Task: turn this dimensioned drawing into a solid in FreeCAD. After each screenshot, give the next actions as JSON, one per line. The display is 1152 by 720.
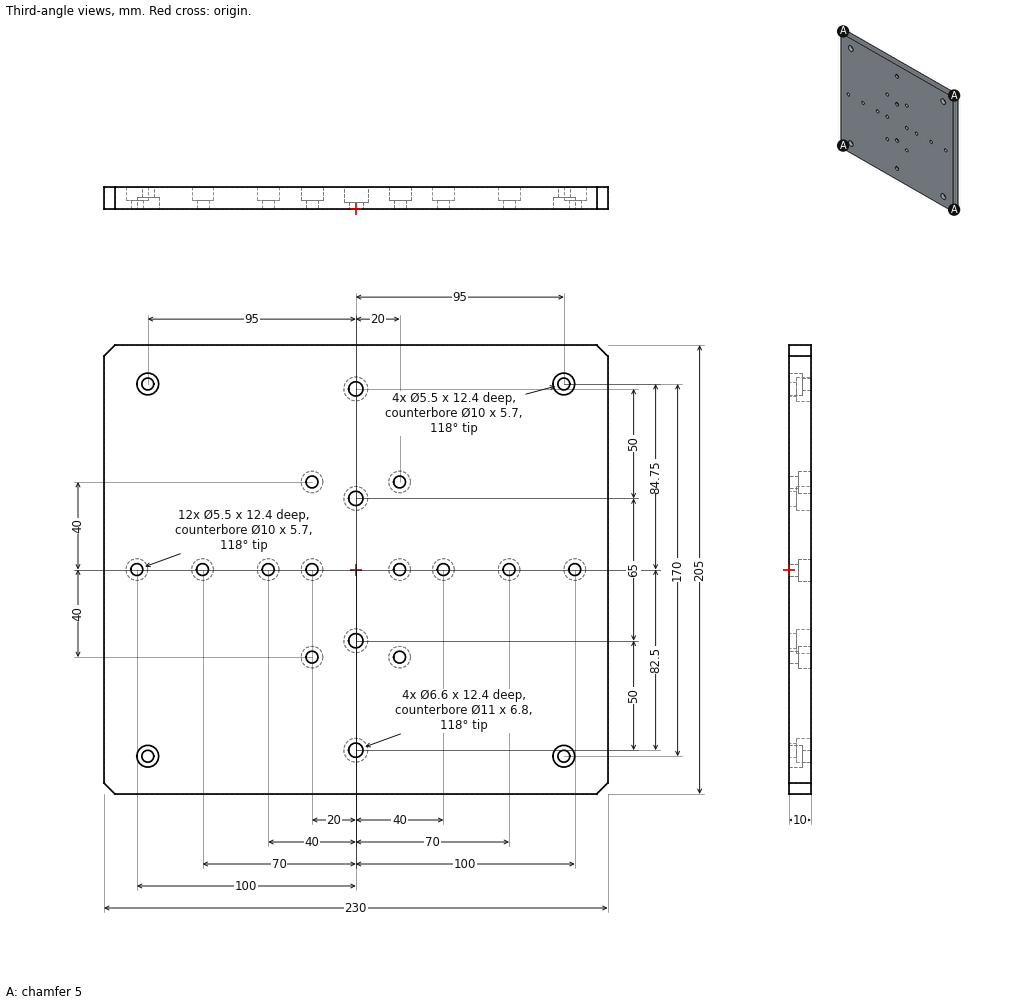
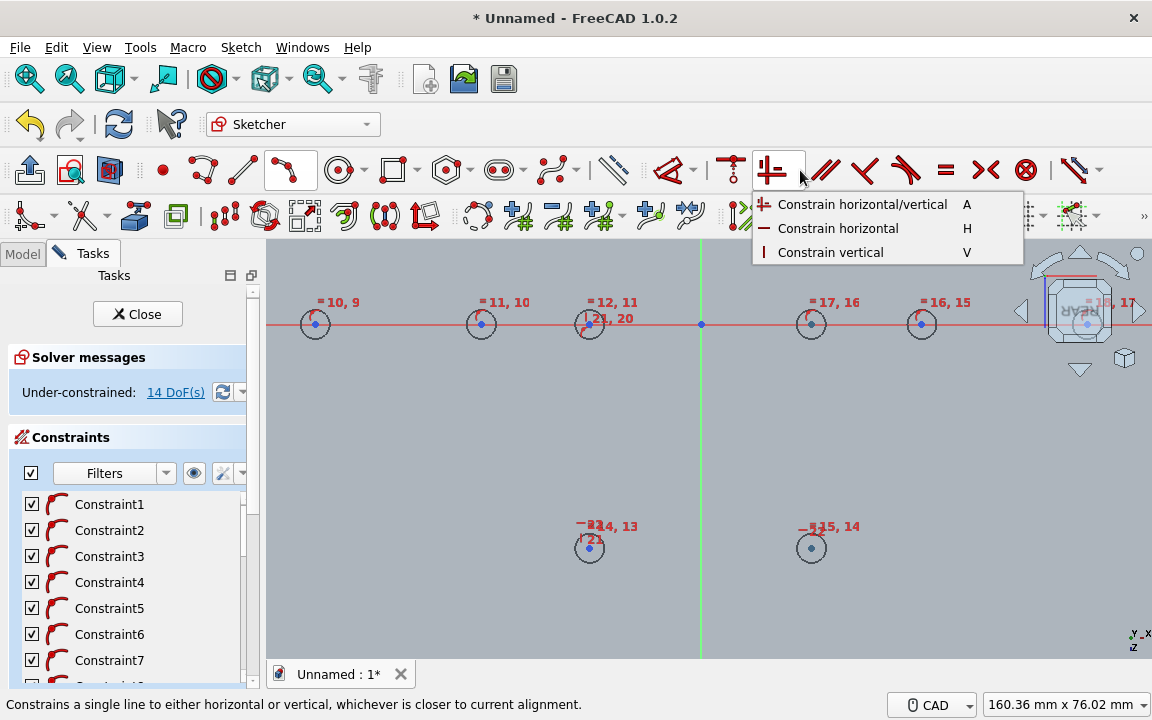
{"action": "left_click", "coordinate": [888, 252]}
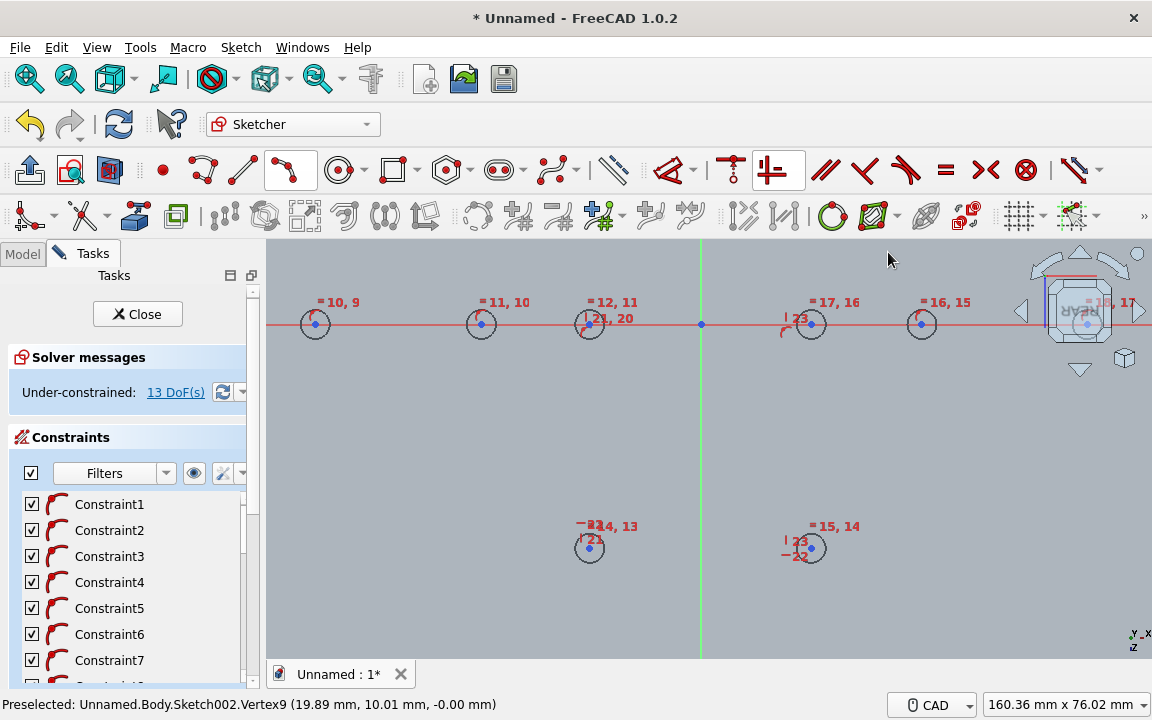
{"action": "left_click", "coordinate": [811, 325]}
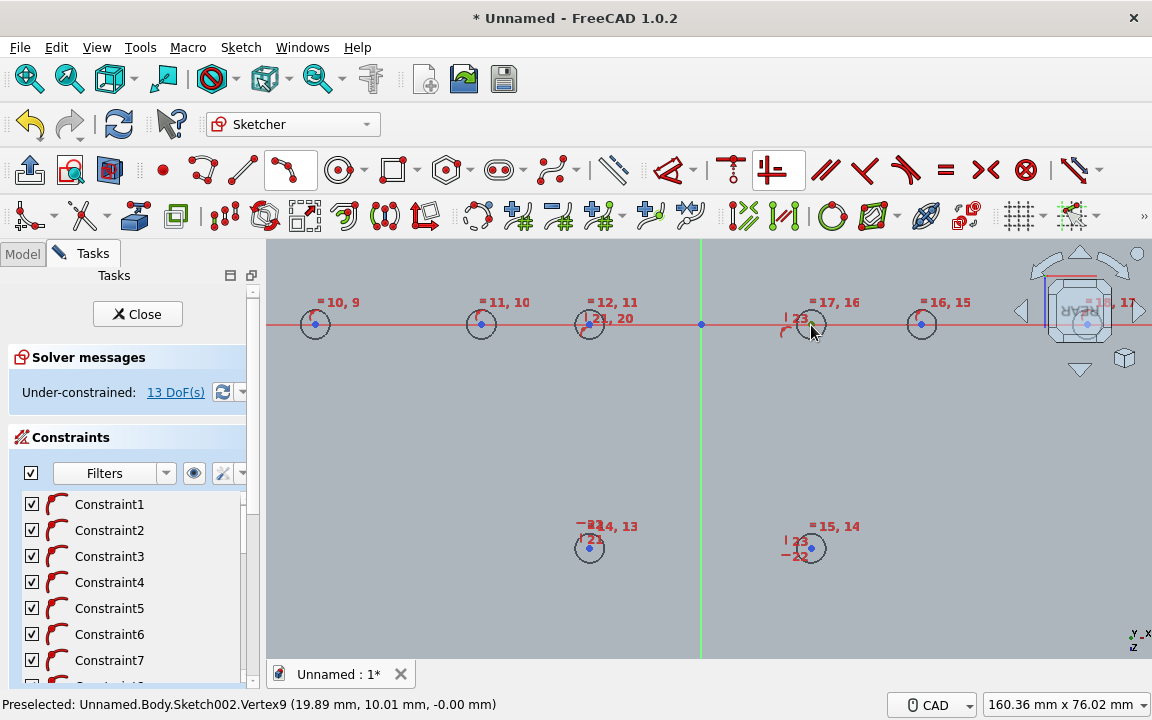
{"action": "scroll", "coordinate": [591, 551], "scroll_direction": "down", "scroll_amount": 4}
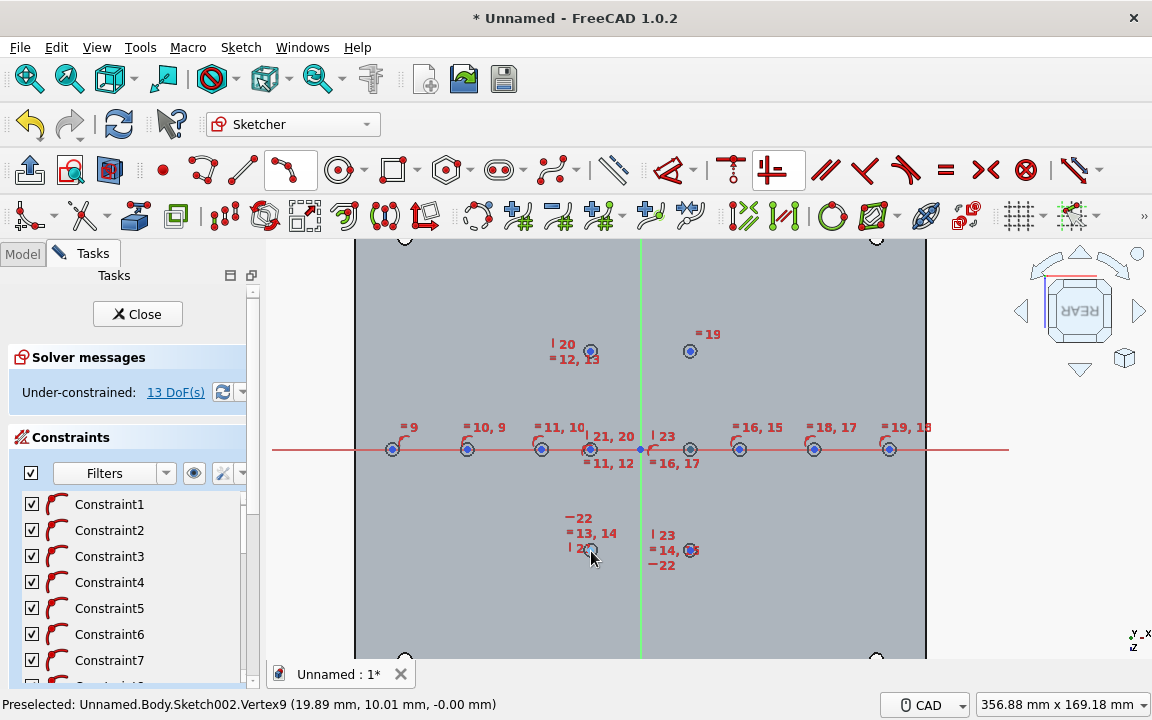
{"action": "left_click", "coordinate": [690, 351]}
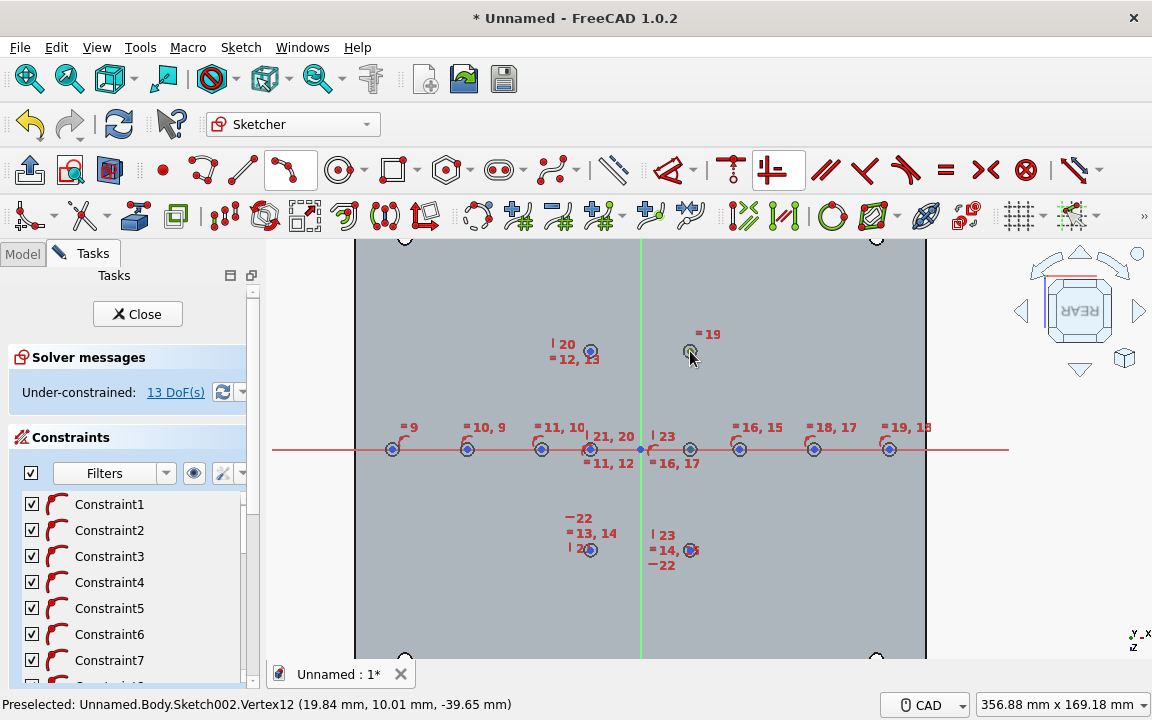
{"action": "key", "text": "v"}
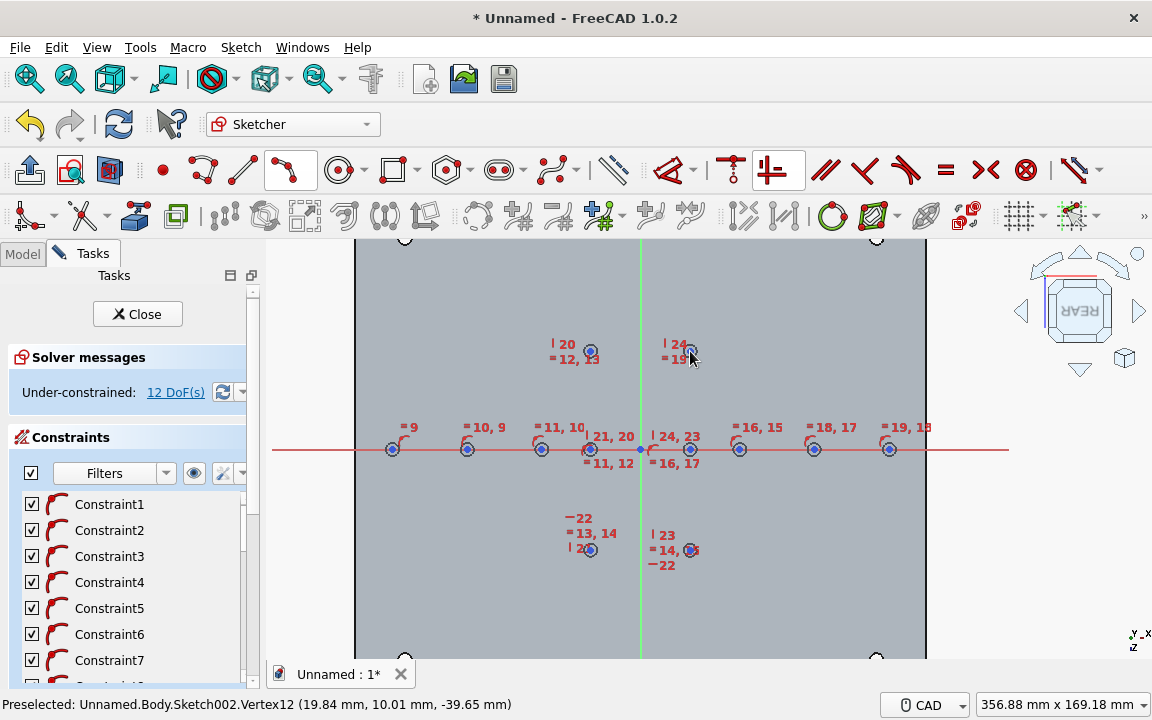
{"action": "scroll", "coordinate": [591, 351], "scroll_direction": "up", "scroll_amount": 4}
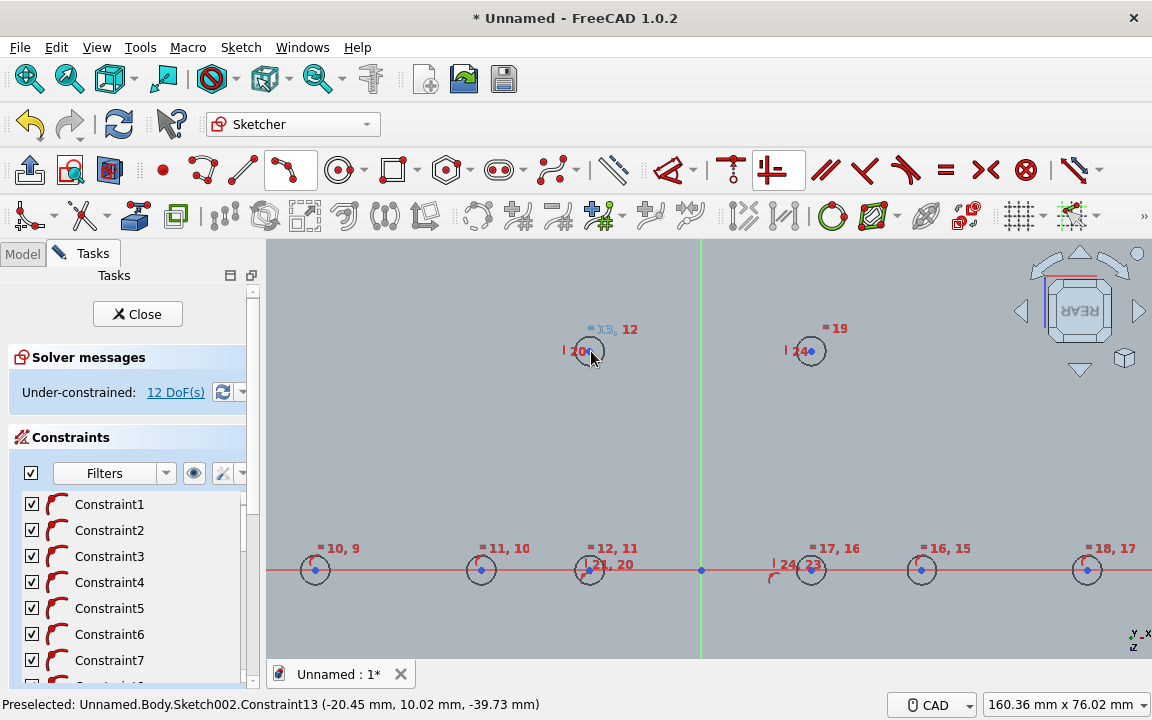
{"action": "left_click", "coordinate": [590, 351]}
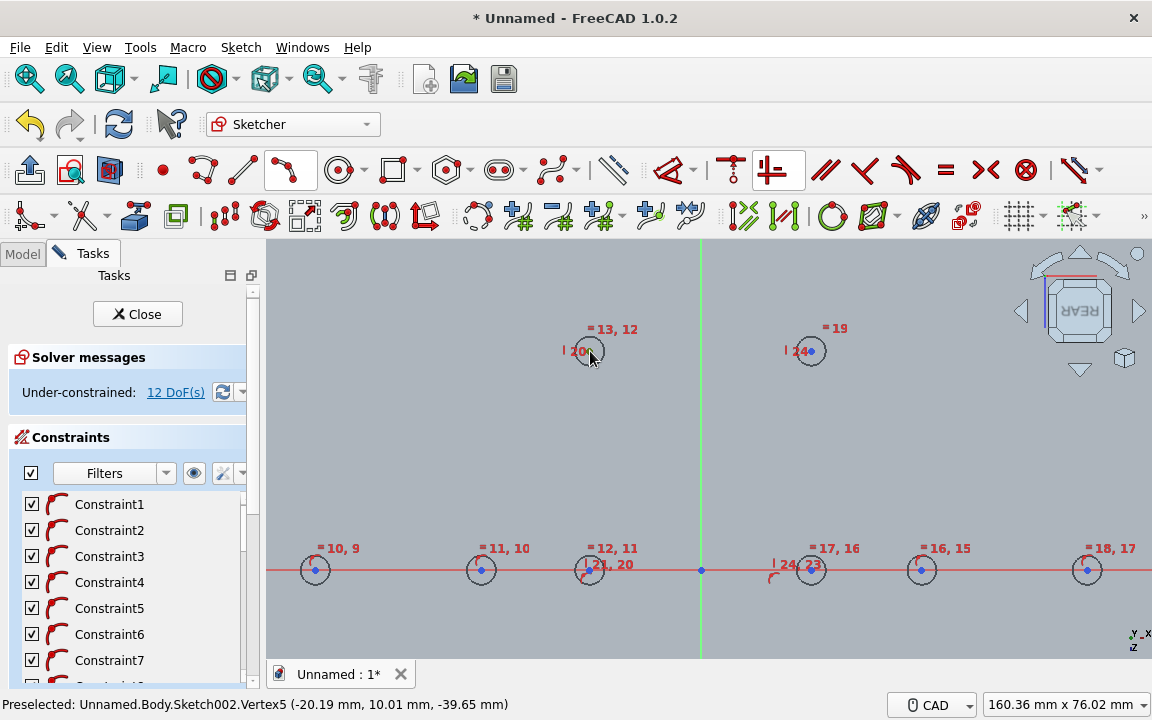
{"action": "left_click", "coordinate": [811, 351]}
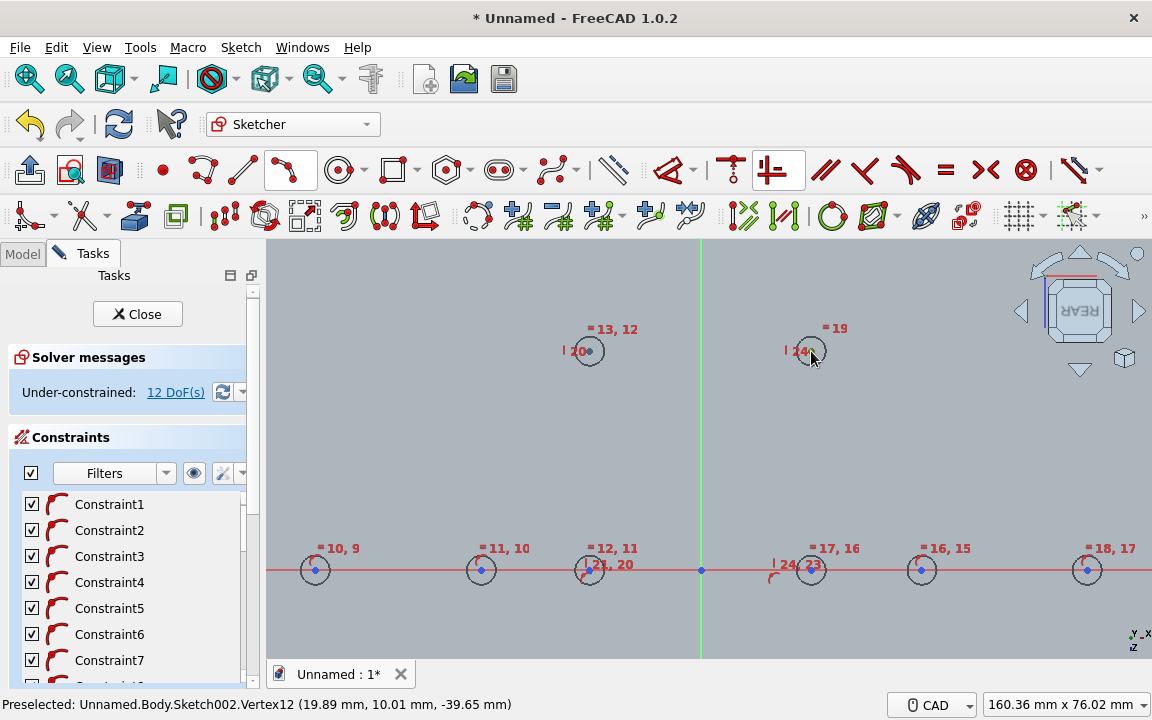
{"action": "key", "text": "h"}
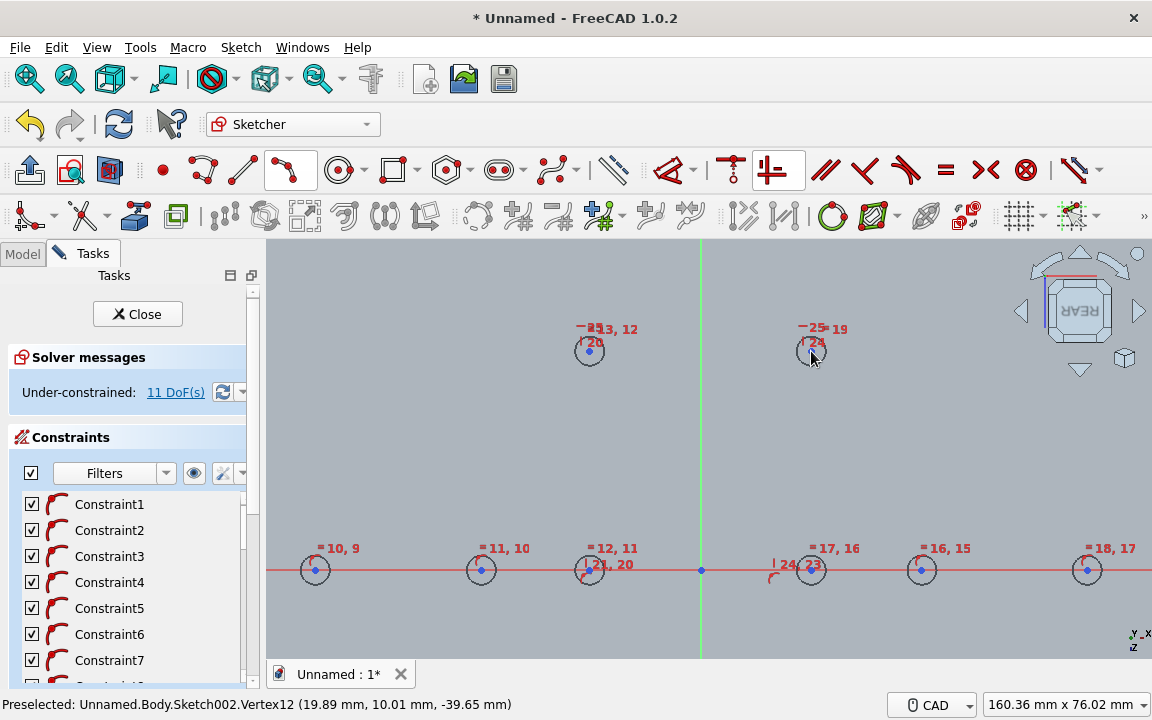
{"action": "left_click", "coordinate": [668, 170]}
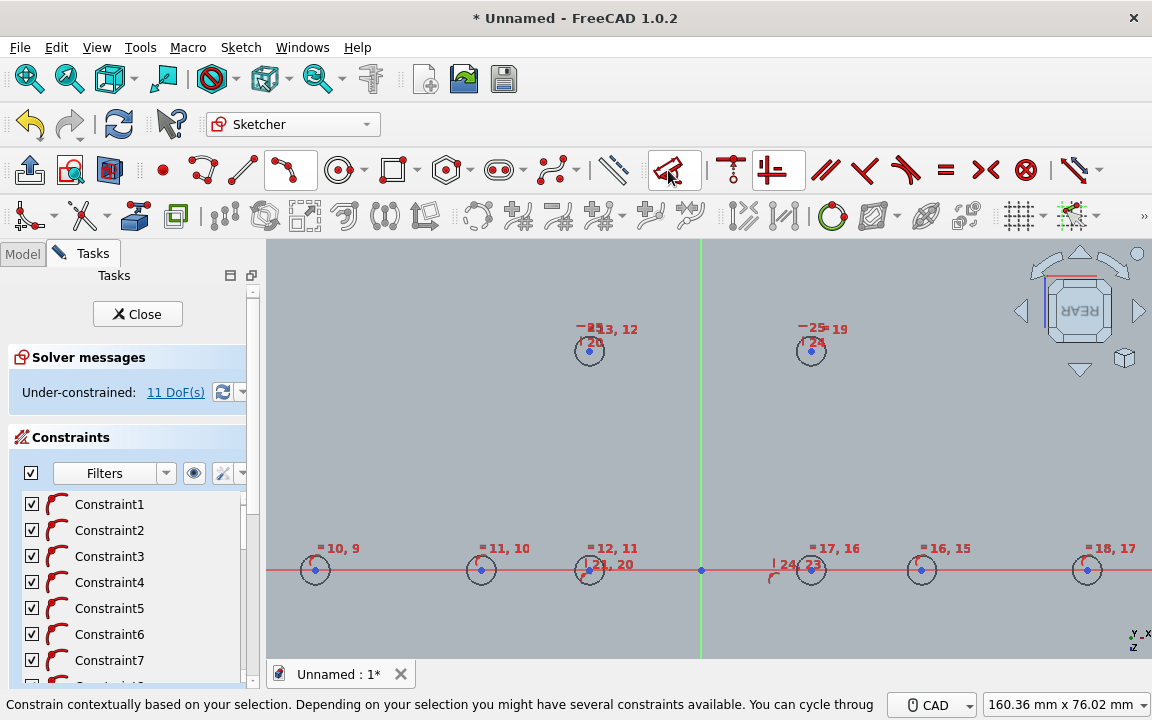
{"action": "scroll", "coordinate": [591, 350], "scroll_direction": "down", "scroll_amount": 4}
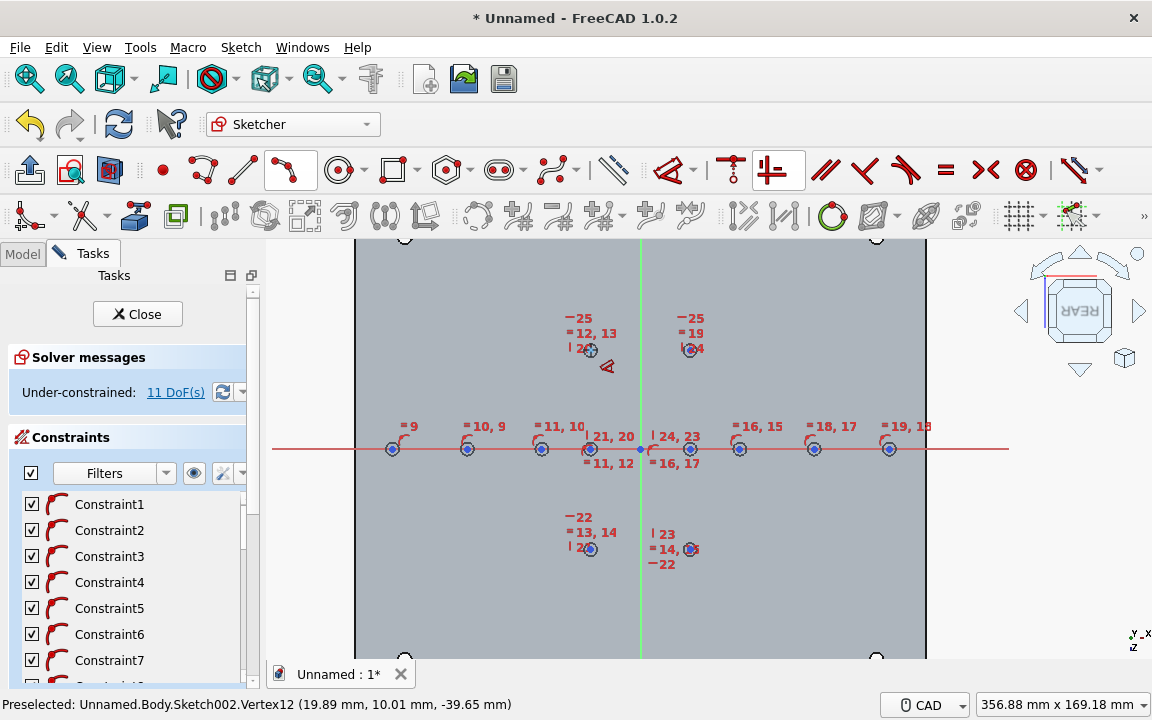
{"action": "scroll", "coordinate": [397, 444], "scroll_direction": "up", "scroll_amount": 6}